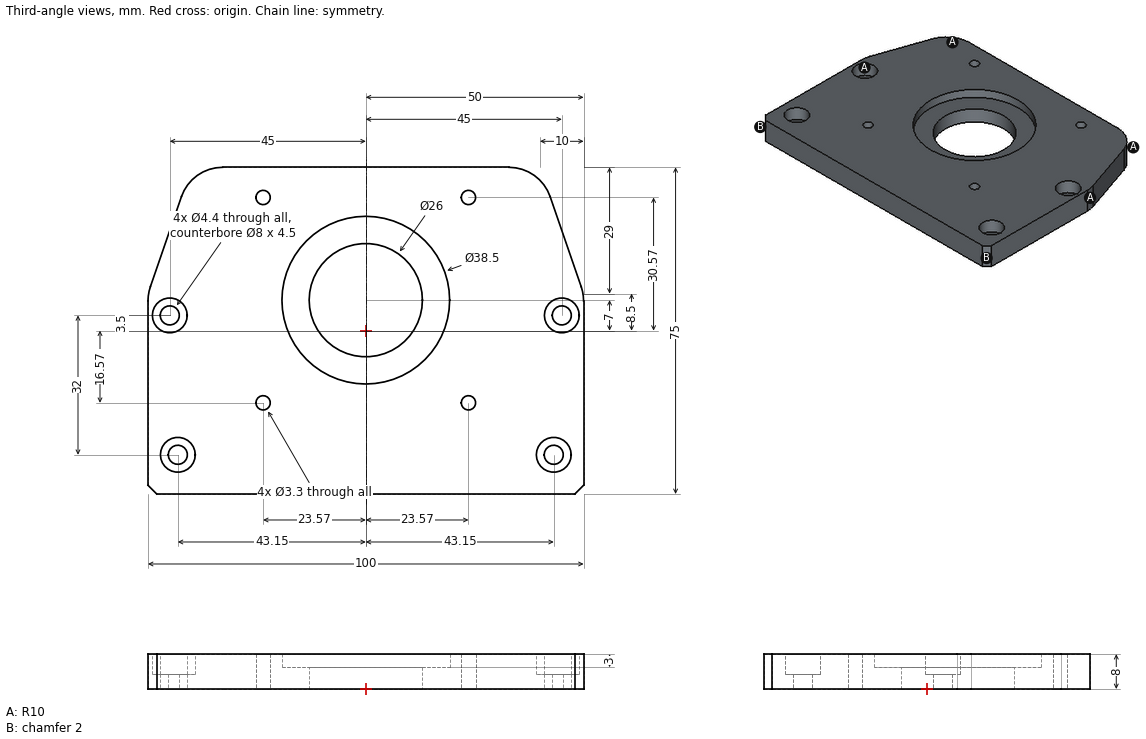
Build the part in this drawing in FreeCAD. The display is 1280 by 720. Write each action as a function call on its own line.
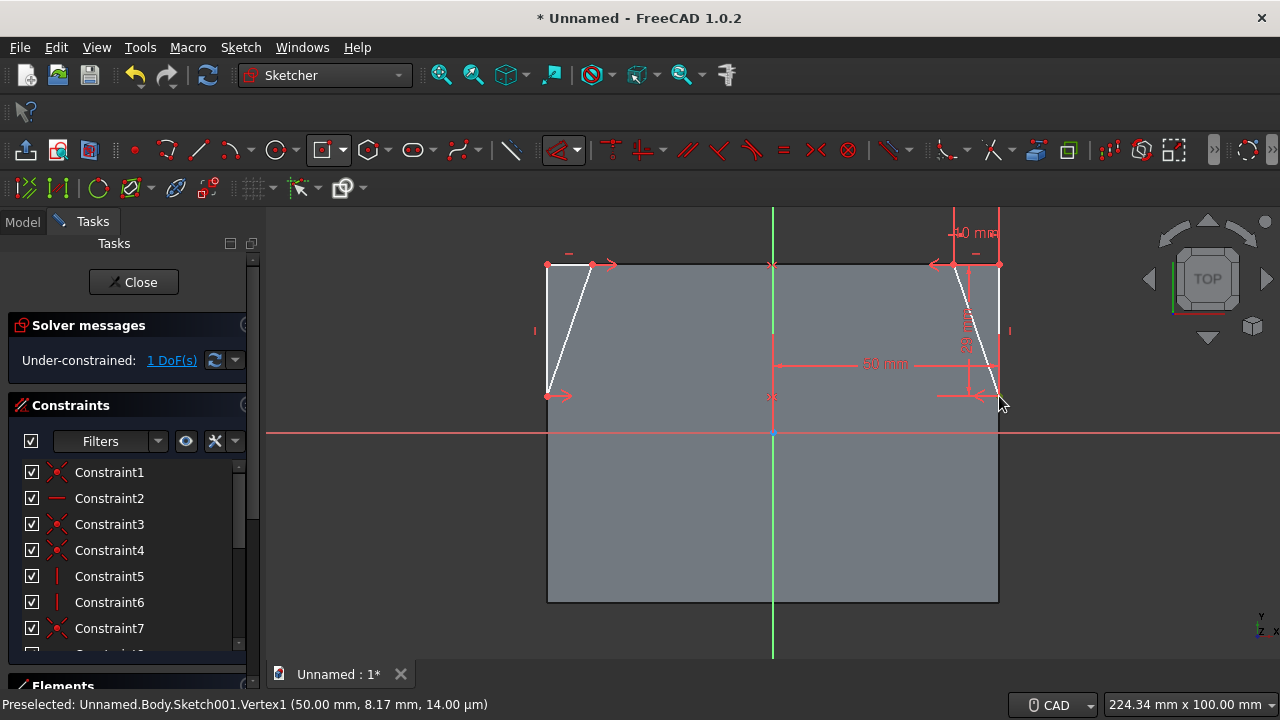
click(580, 150)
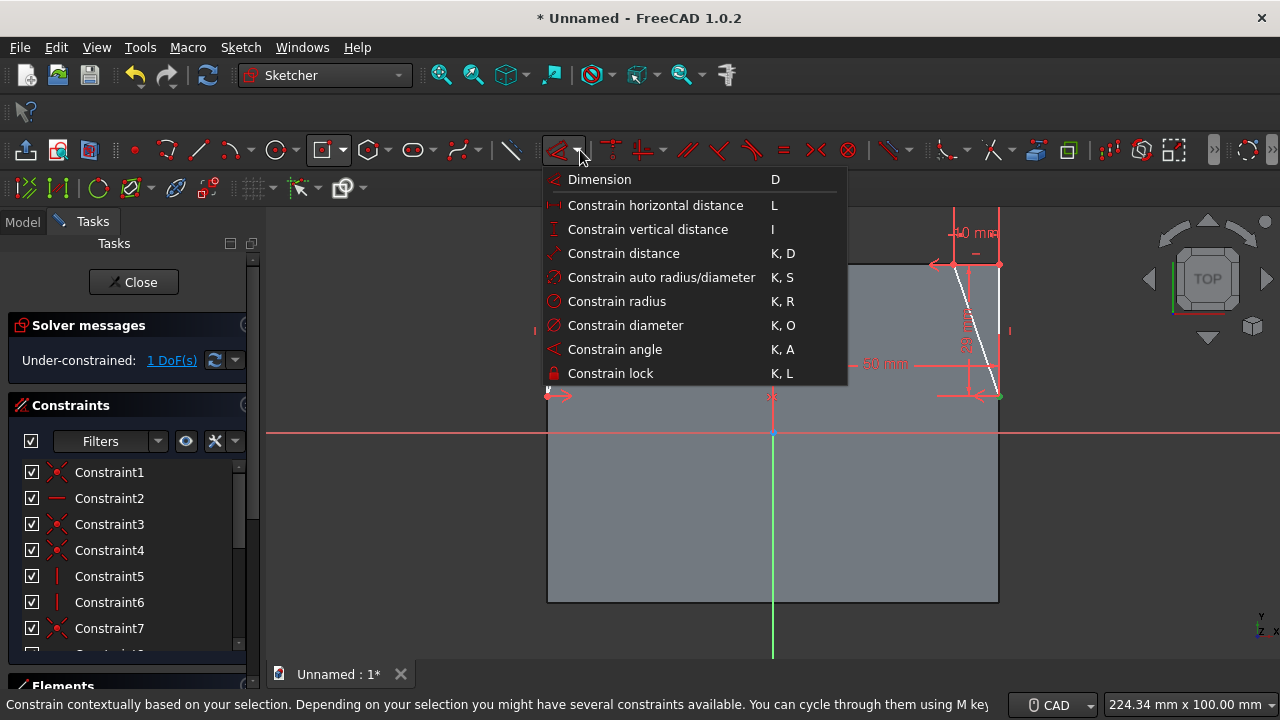
click(695, 229)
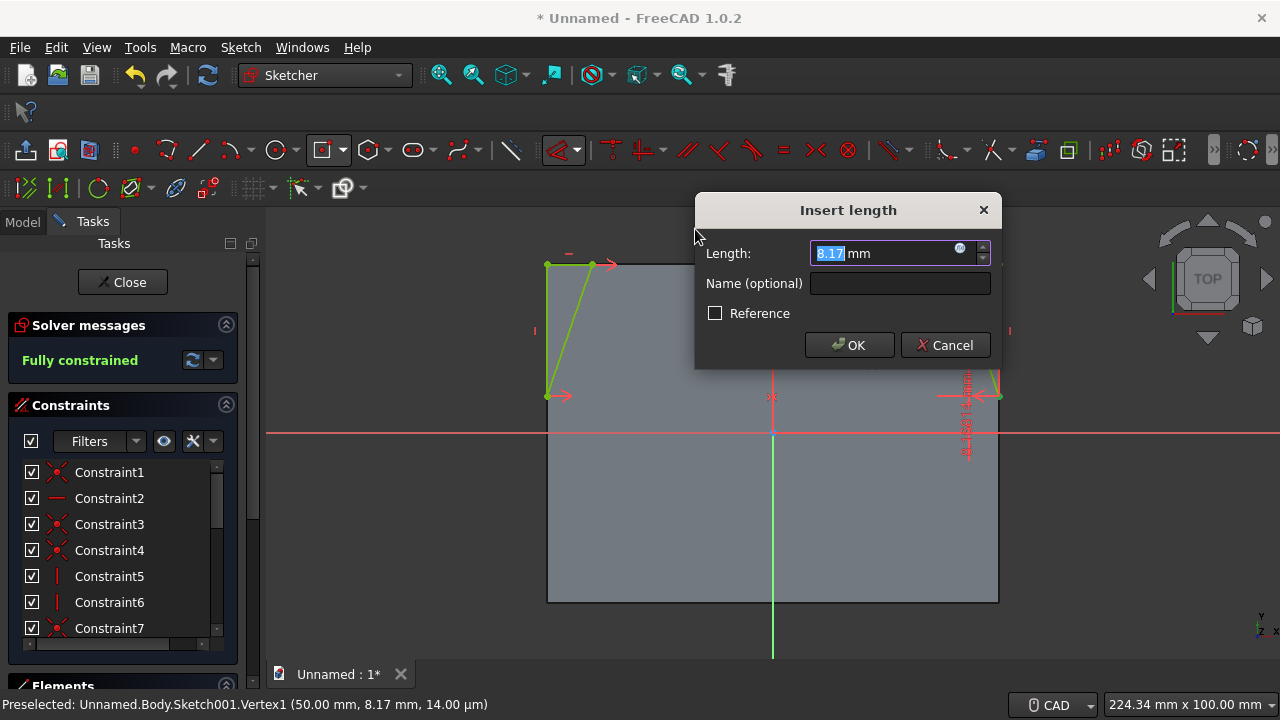
text(8.5)
key(Return)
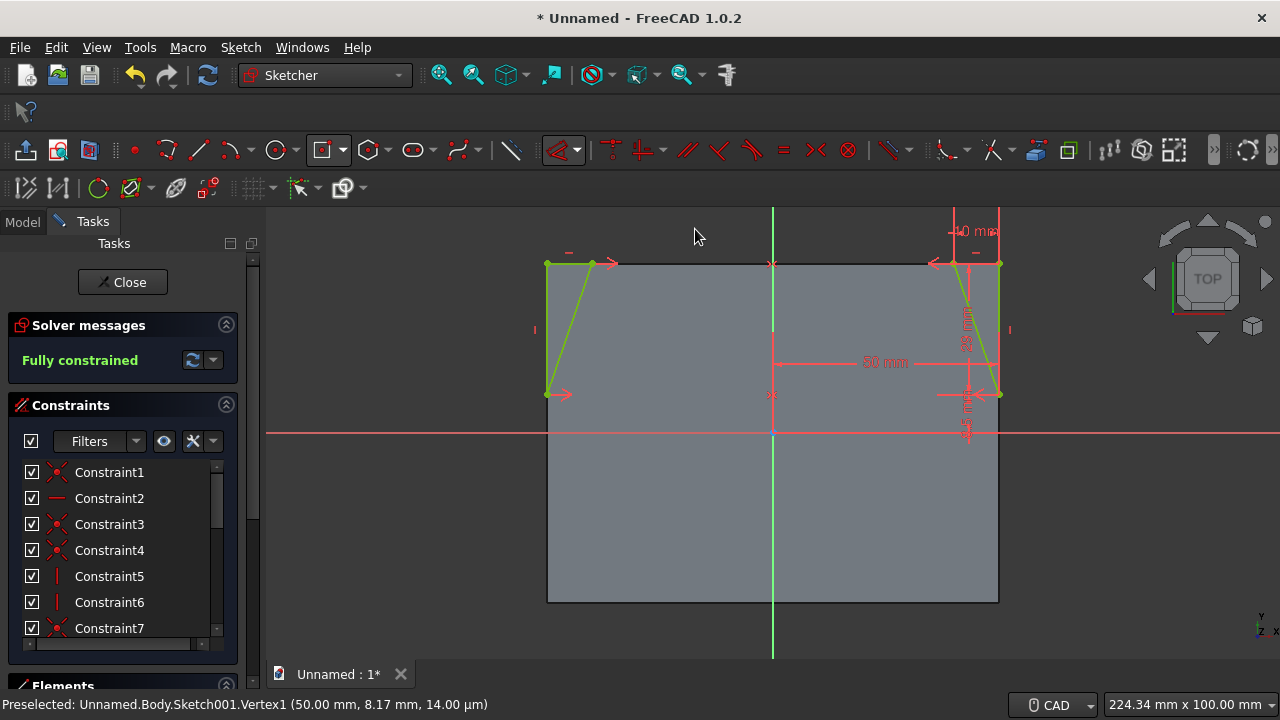
click(123, 282)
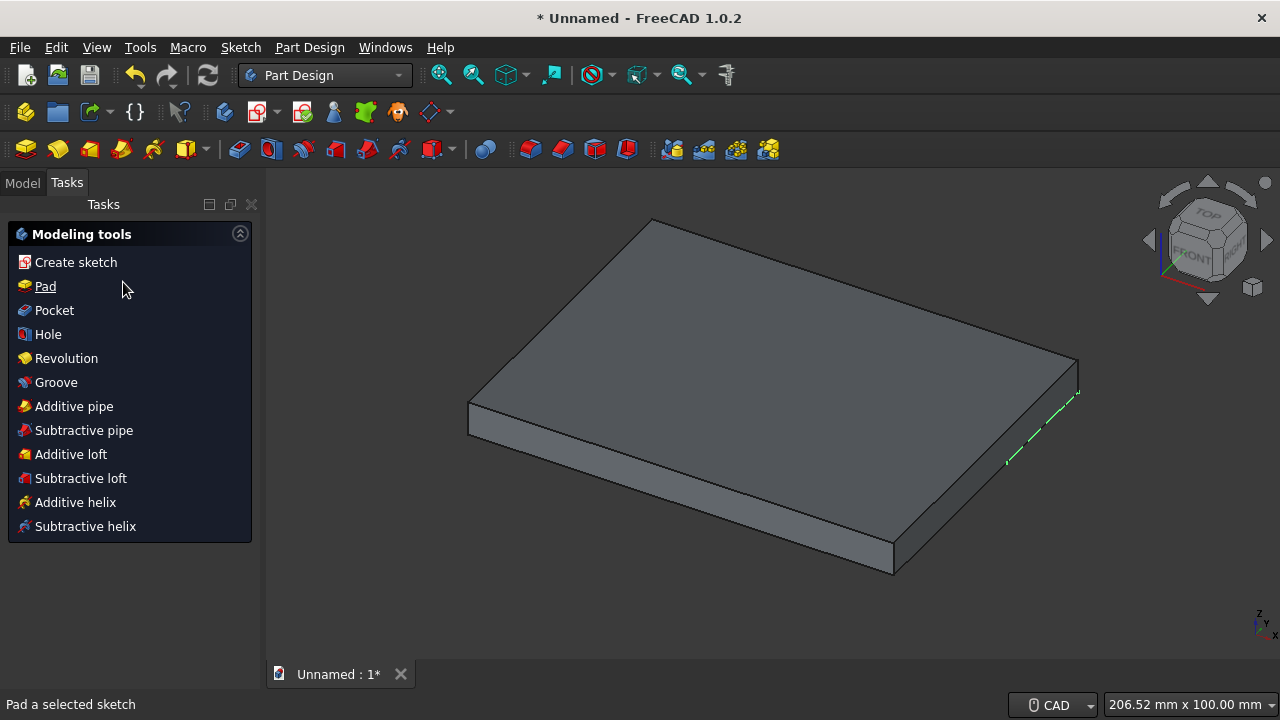
click(240, 150)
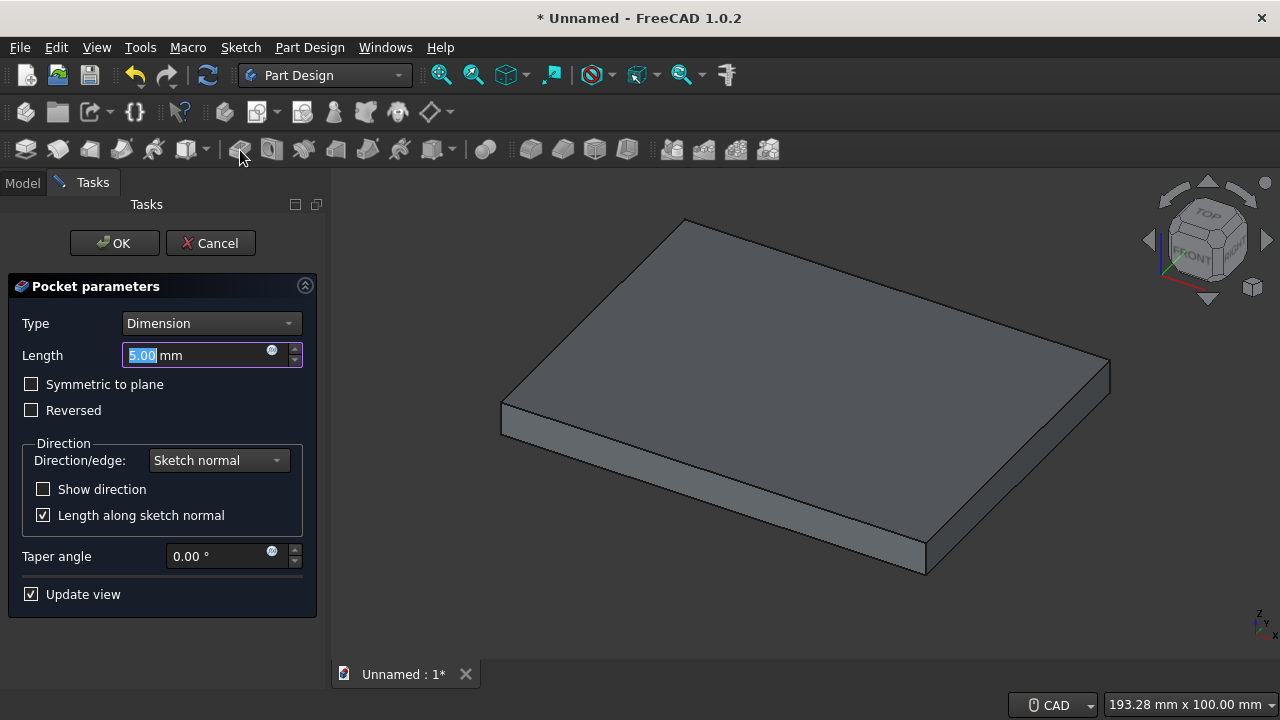
text(10)
key(Tab)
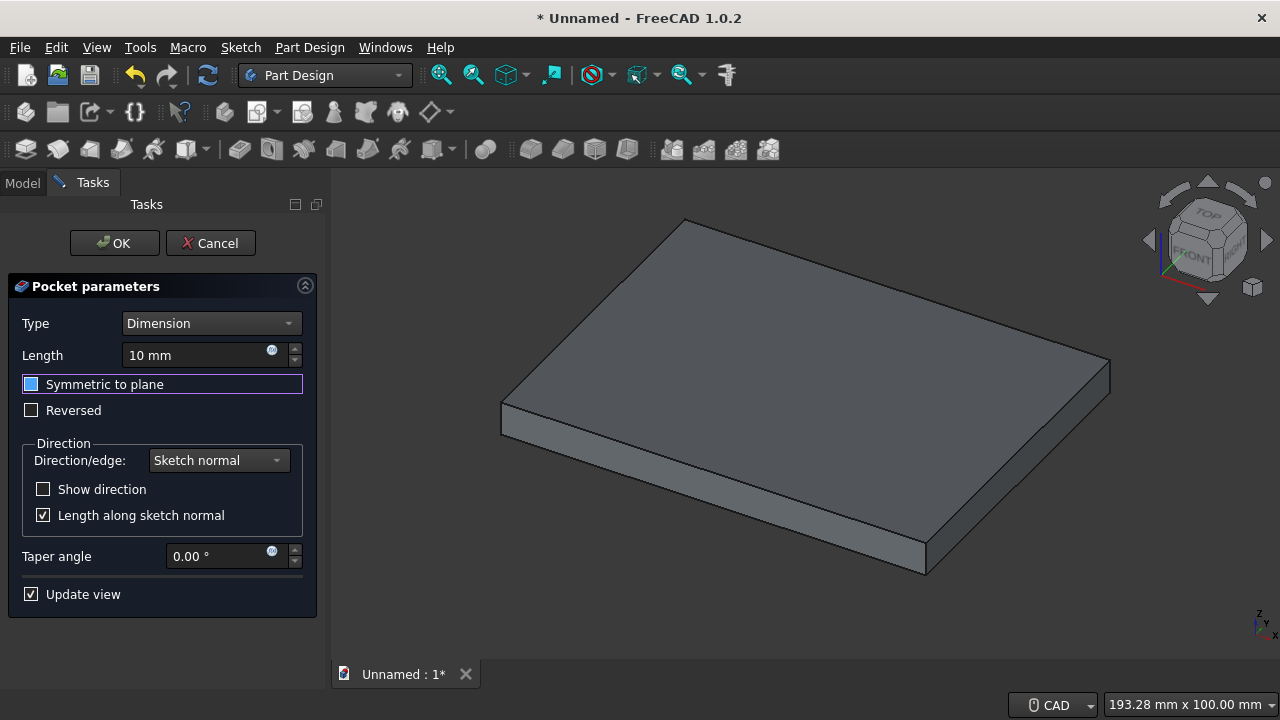
click(30, 410)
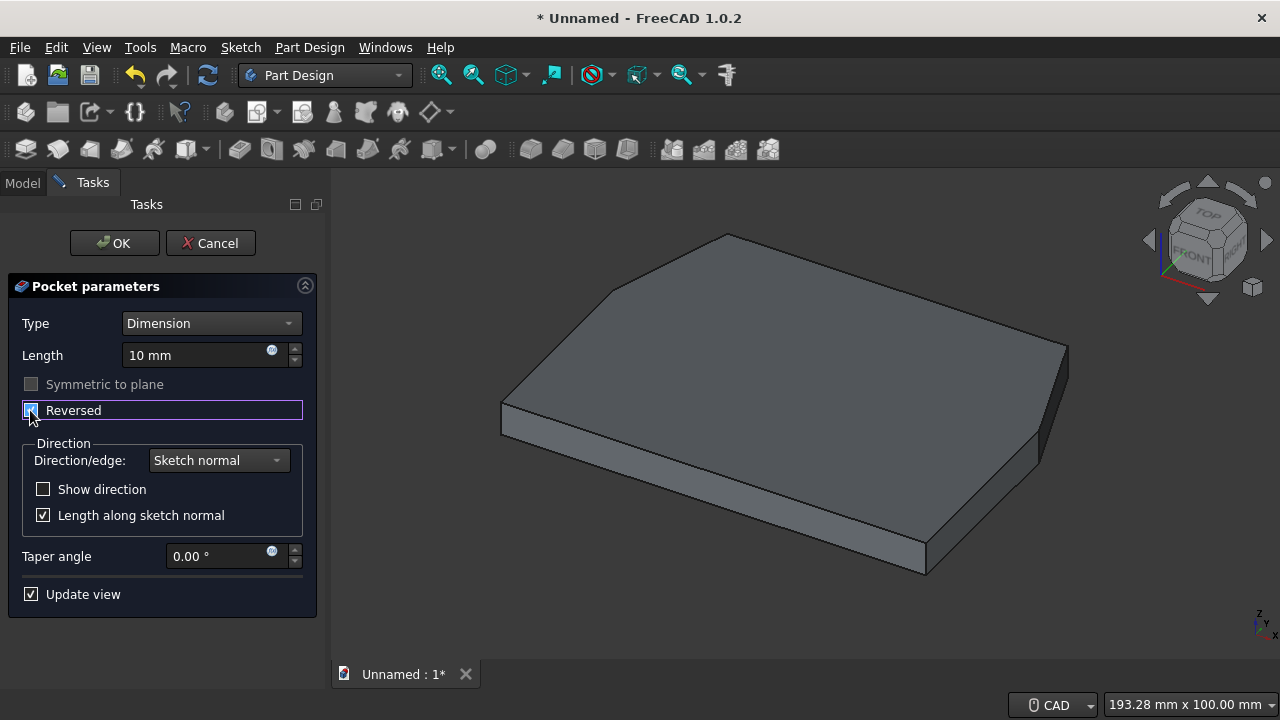
click(115, 243)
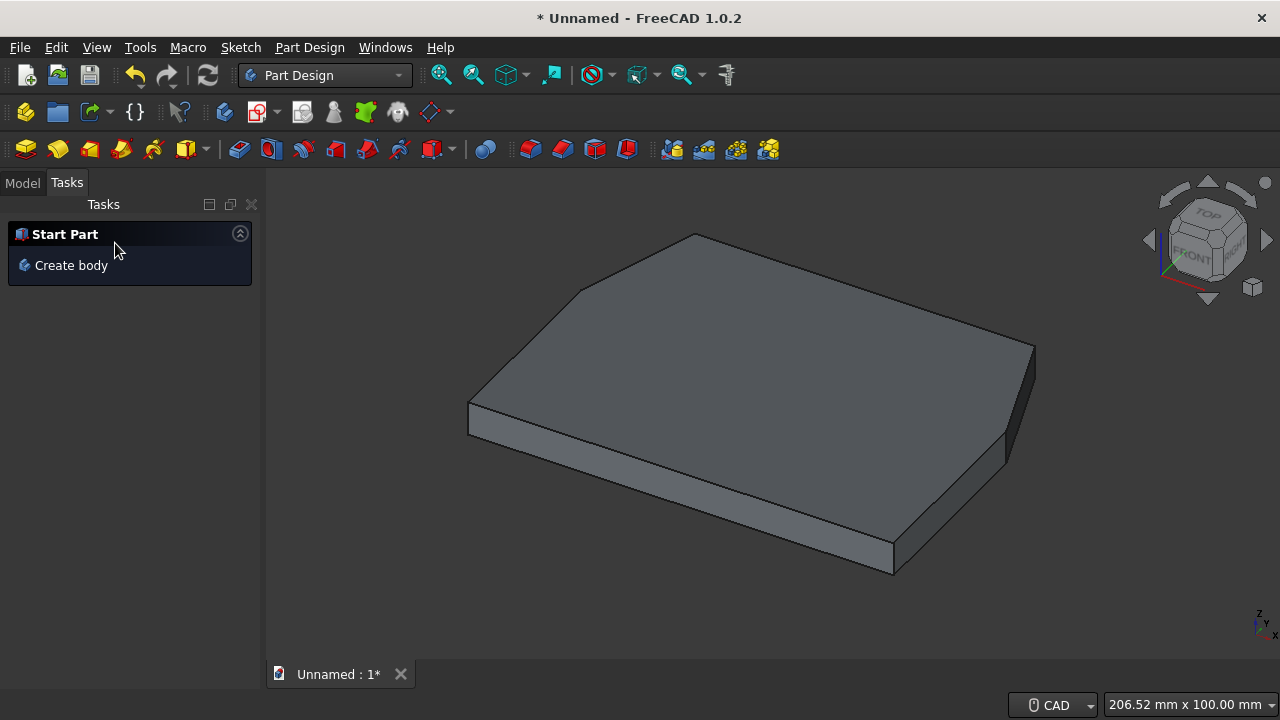
key(0)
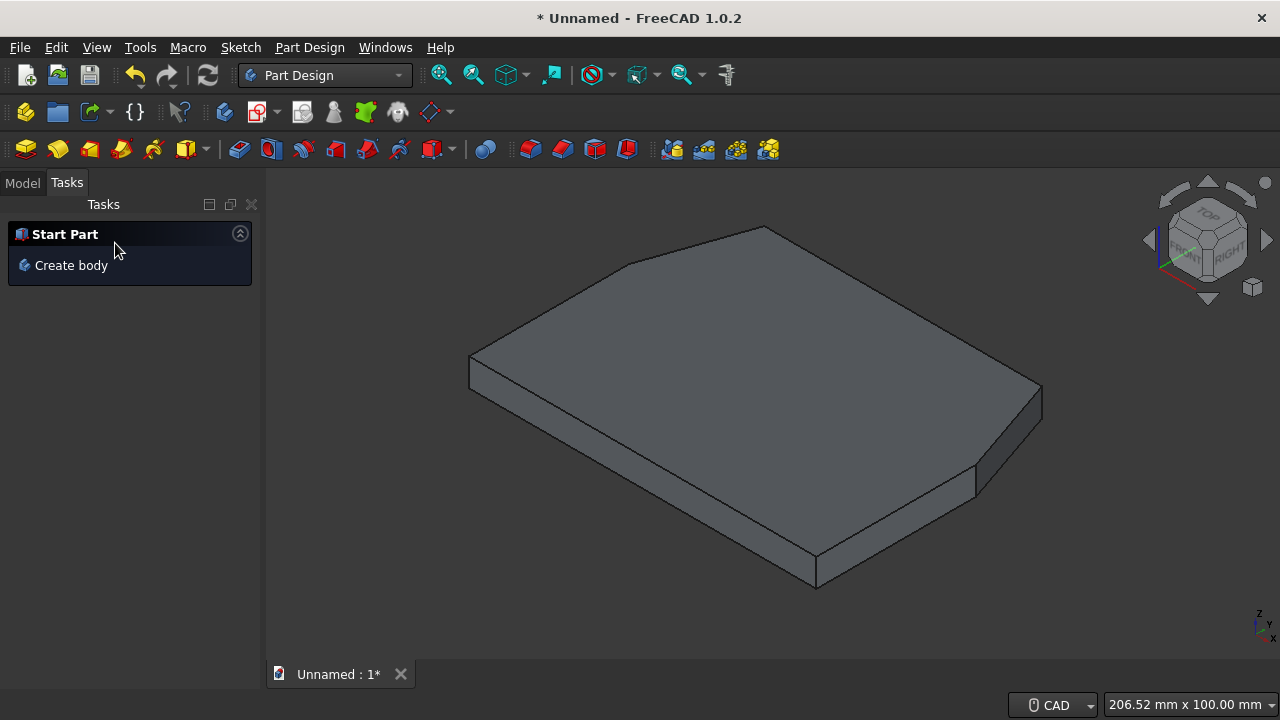
key(2)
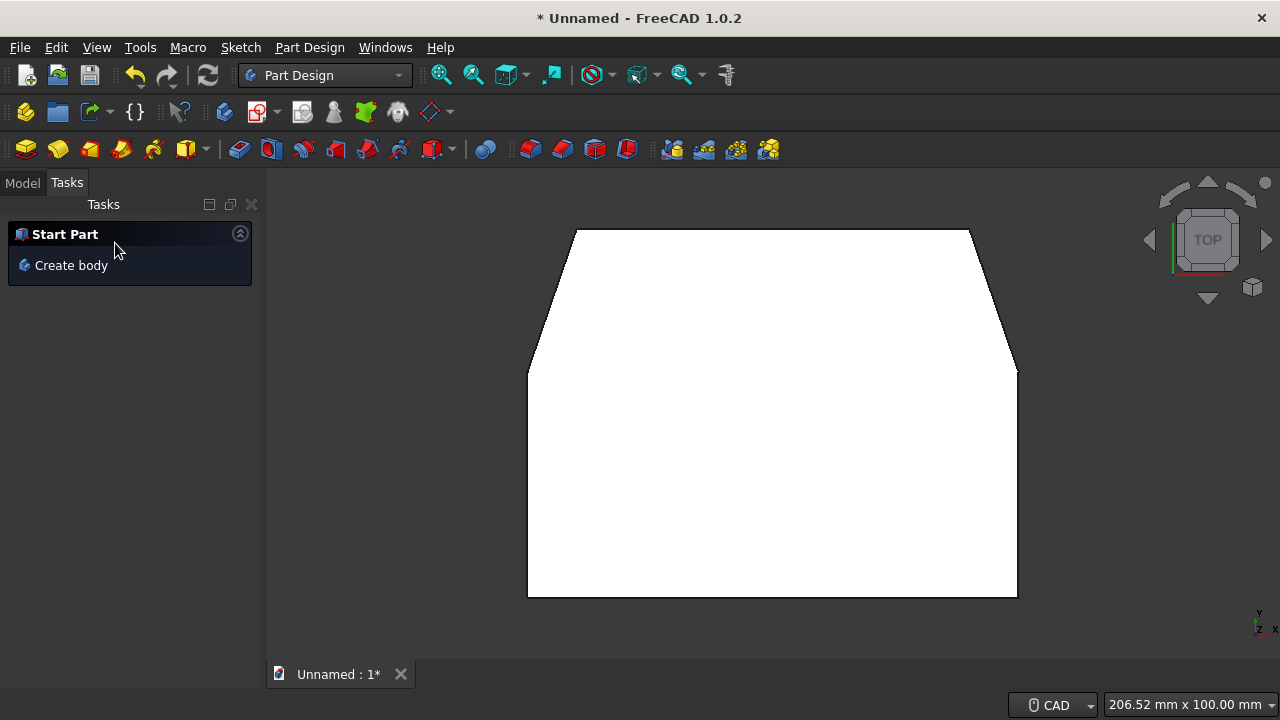
key(1)